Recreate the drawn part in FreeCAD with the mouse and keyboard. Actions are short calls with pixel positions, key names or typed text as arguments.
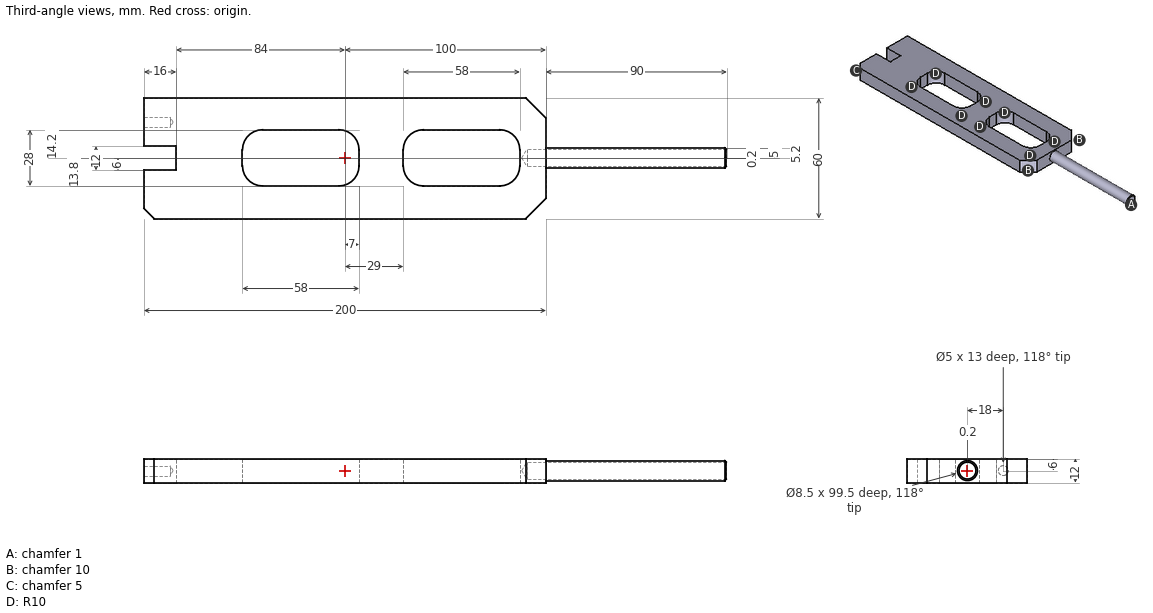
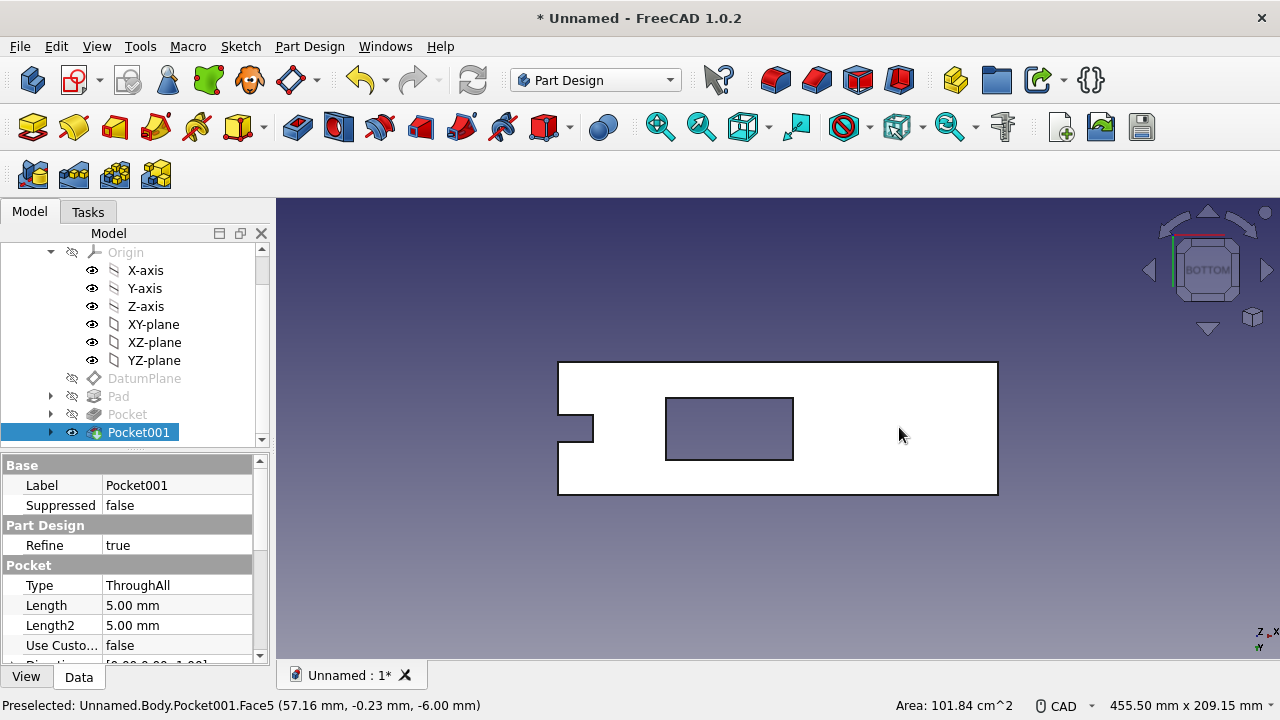
click(74, 80)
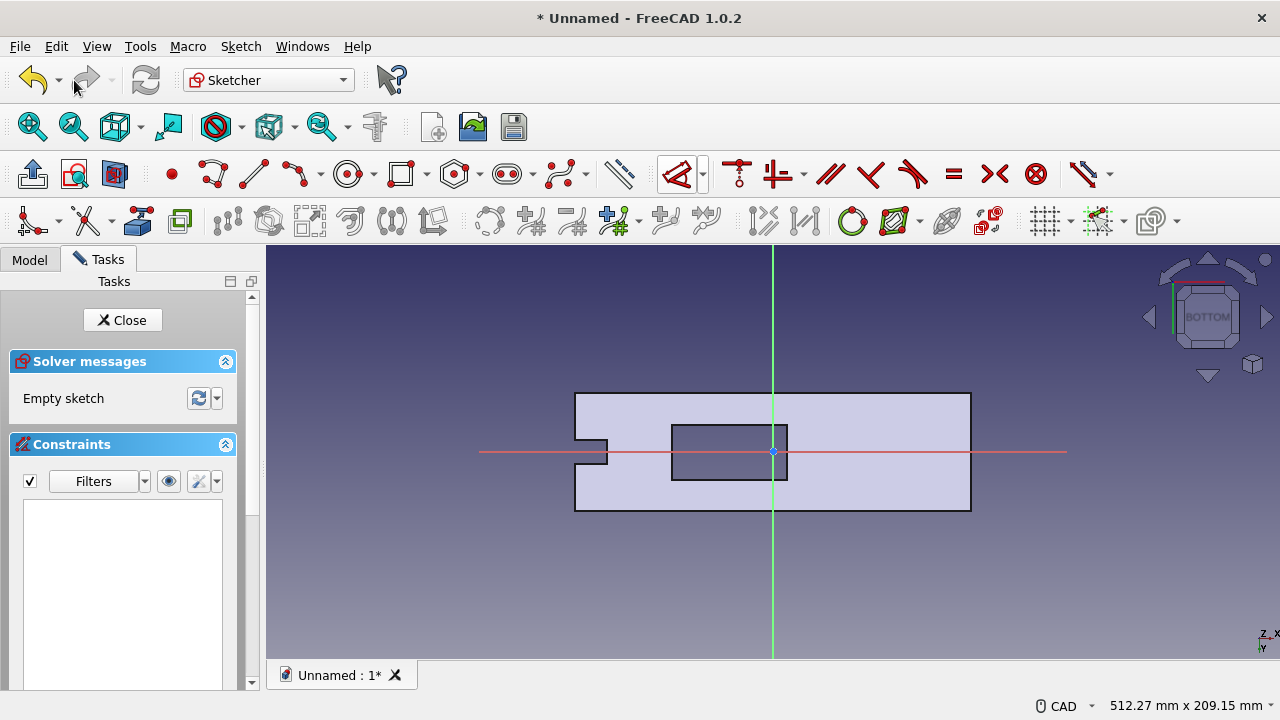
scroll(926, 453, up, 6)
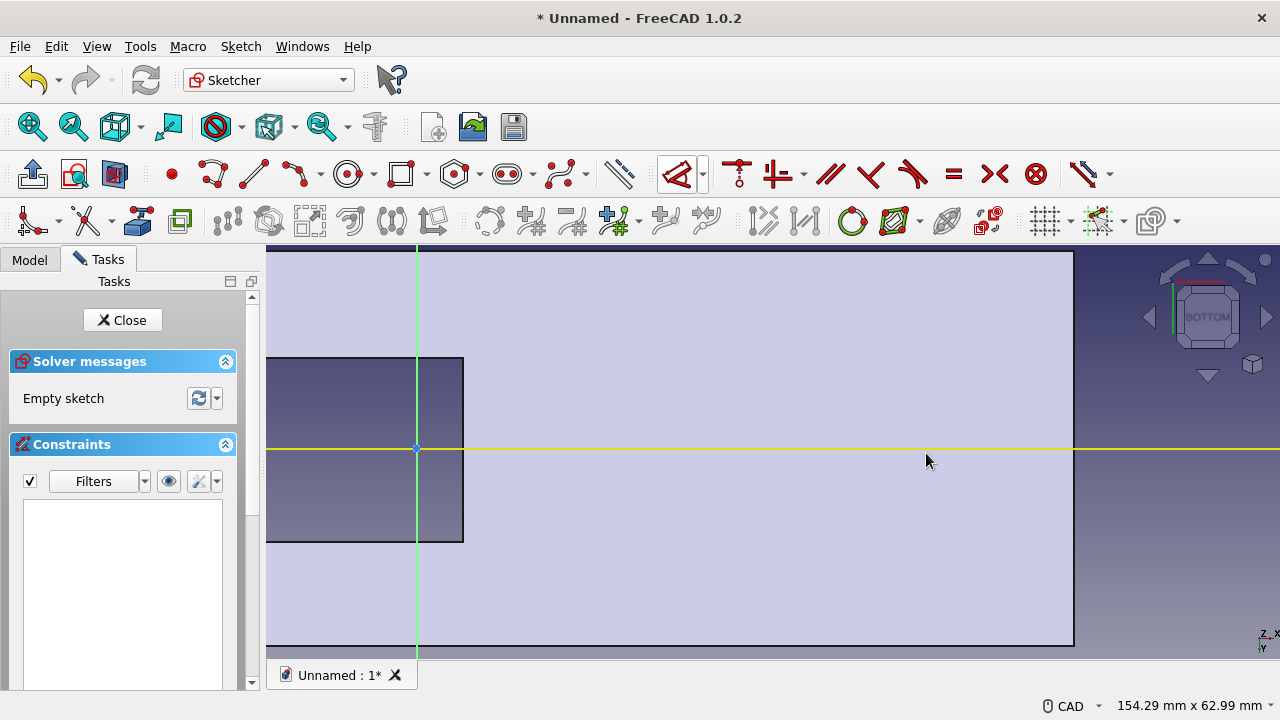
key(g)
key(r)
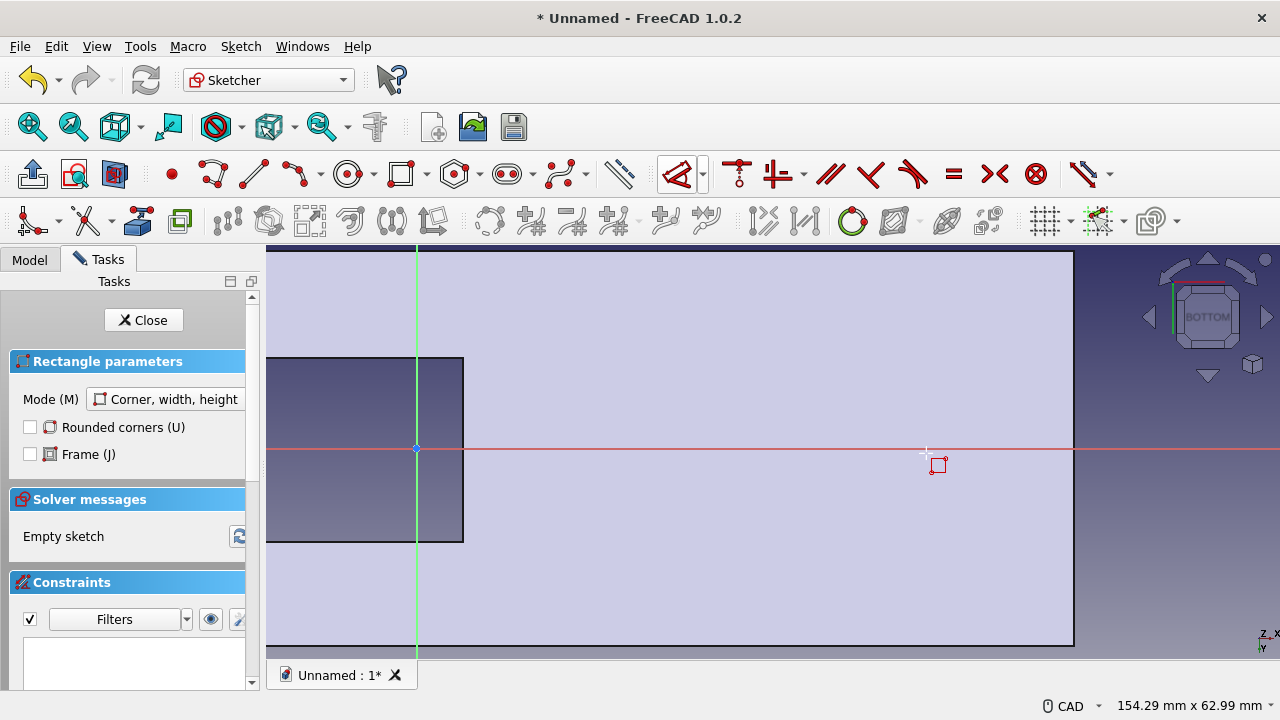
click(607, 358)
move(988, 542)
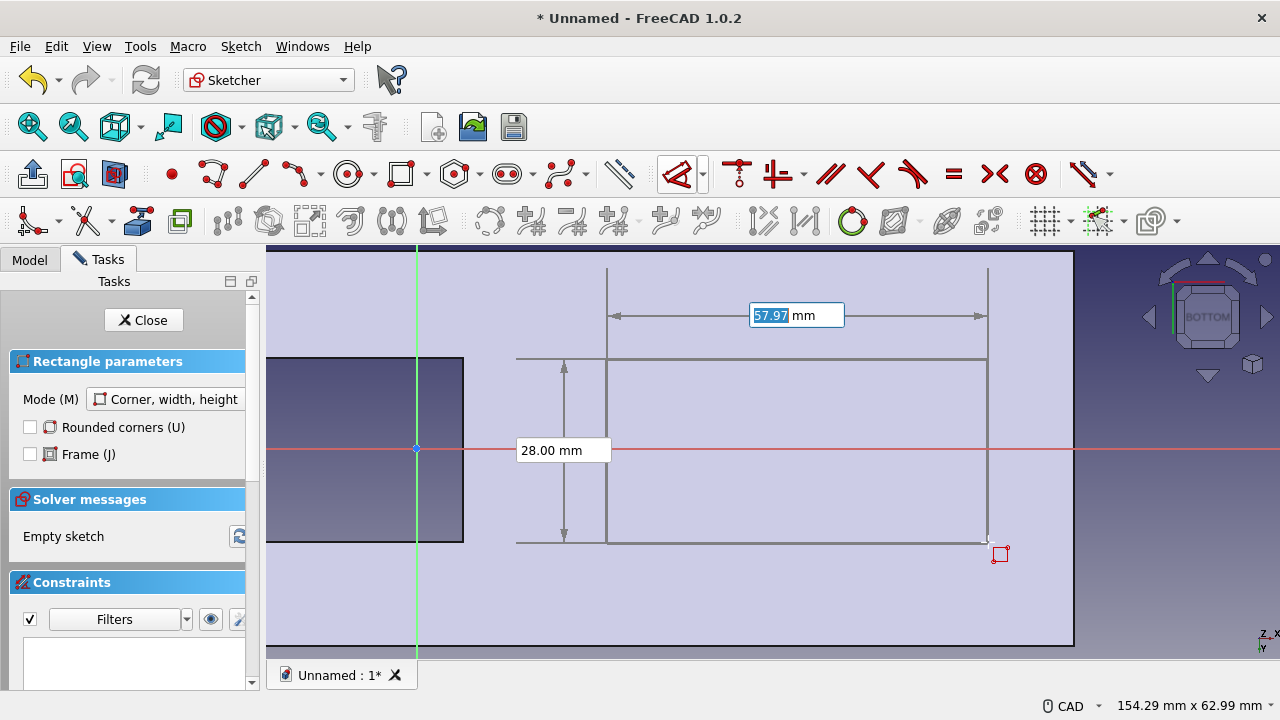
text(58)
key(Tab)
text(28)
key(Return)
key(Escape)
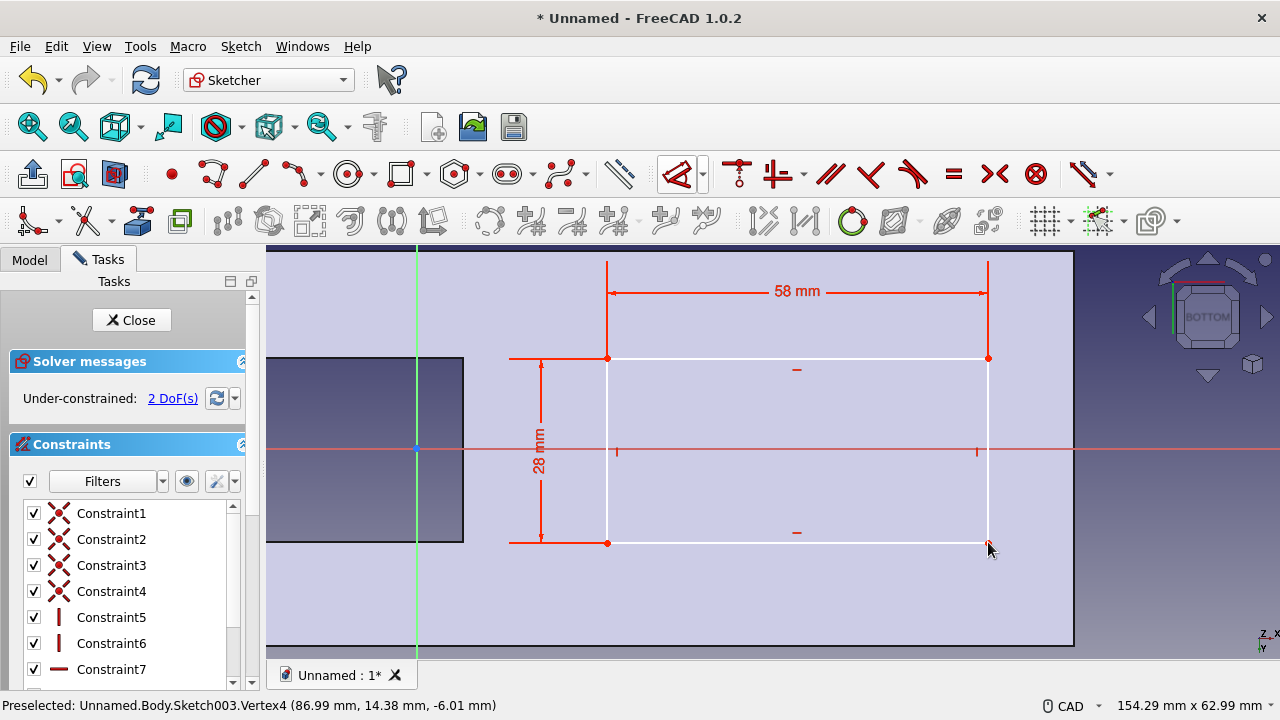
click(607, 359)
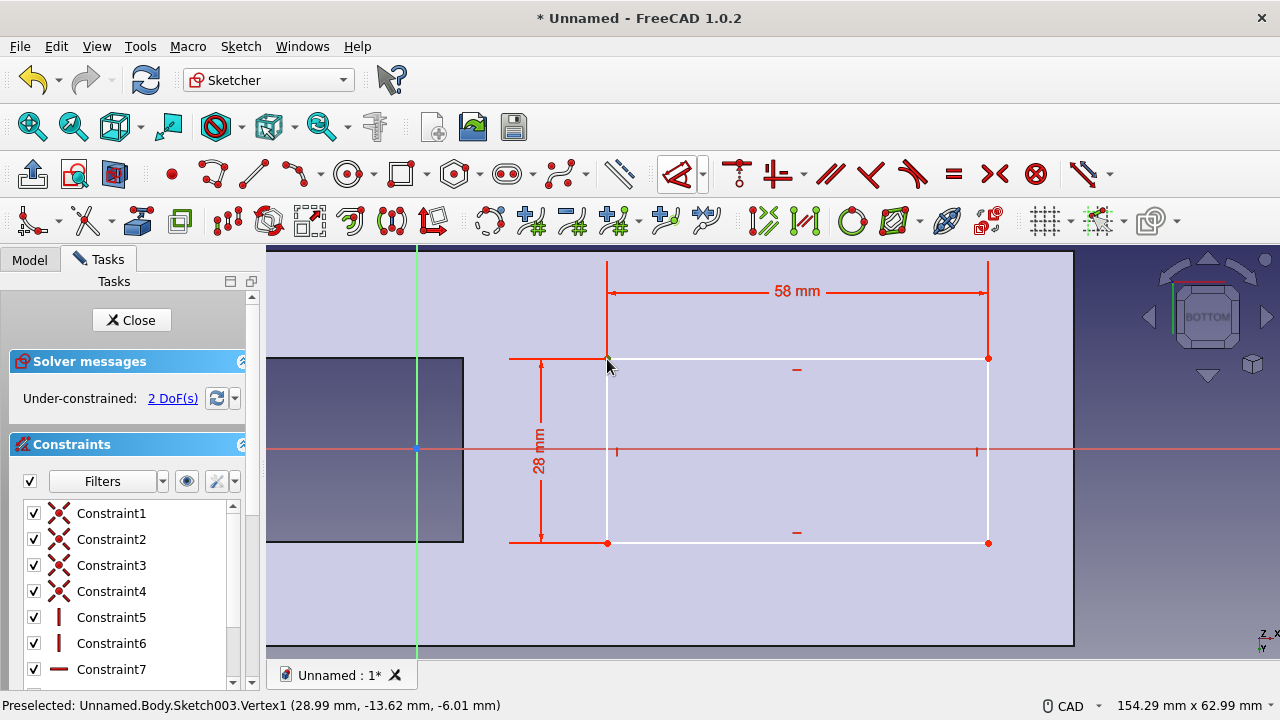
click(702, 174)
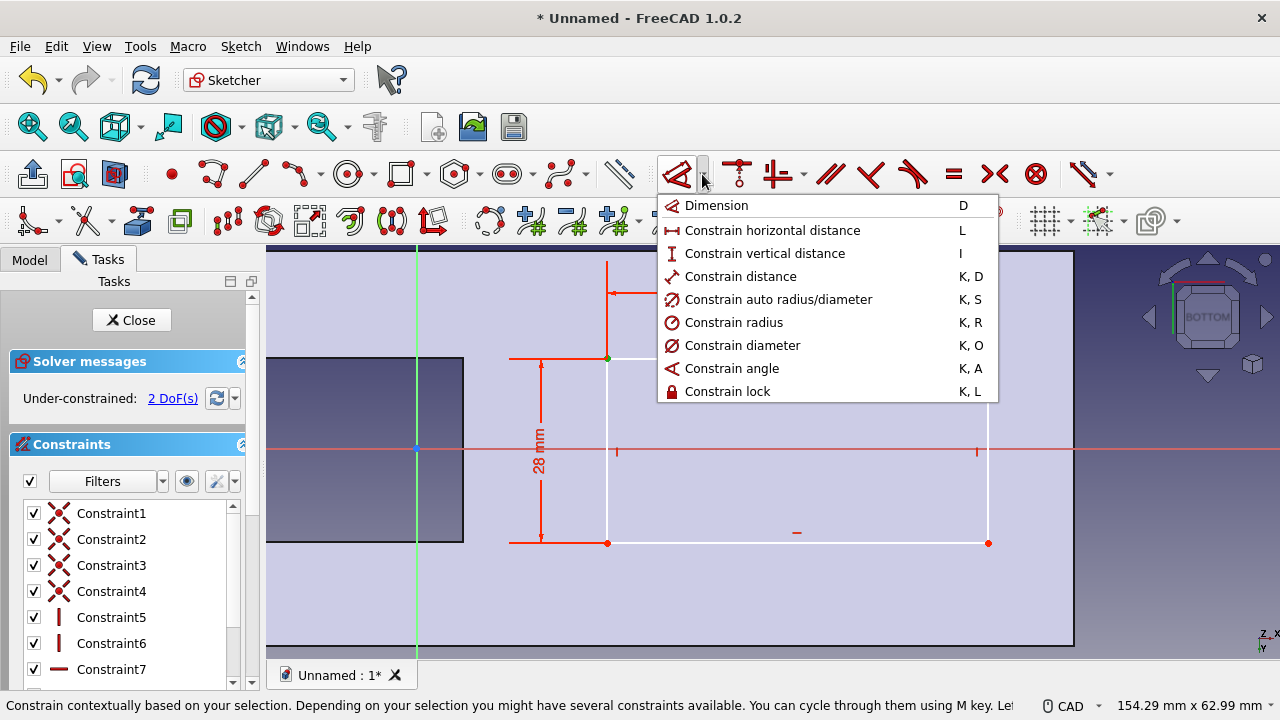
click(828, 230)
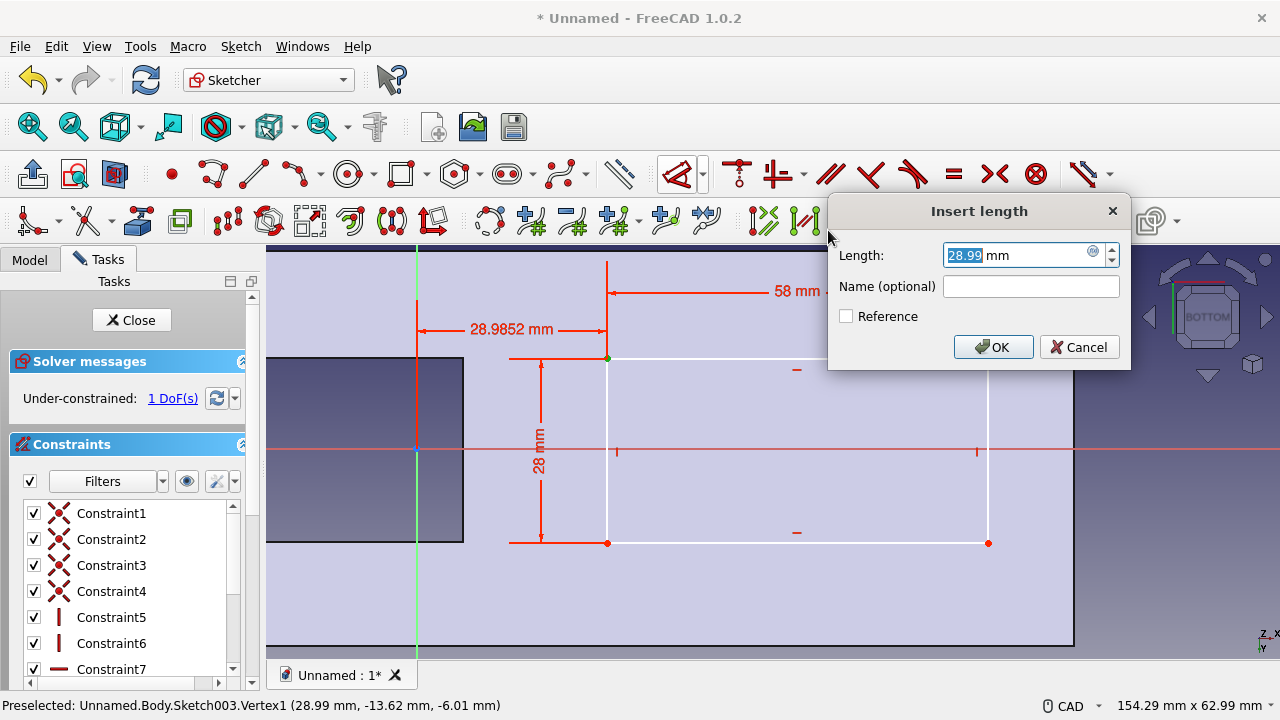
text(29)
key(Return)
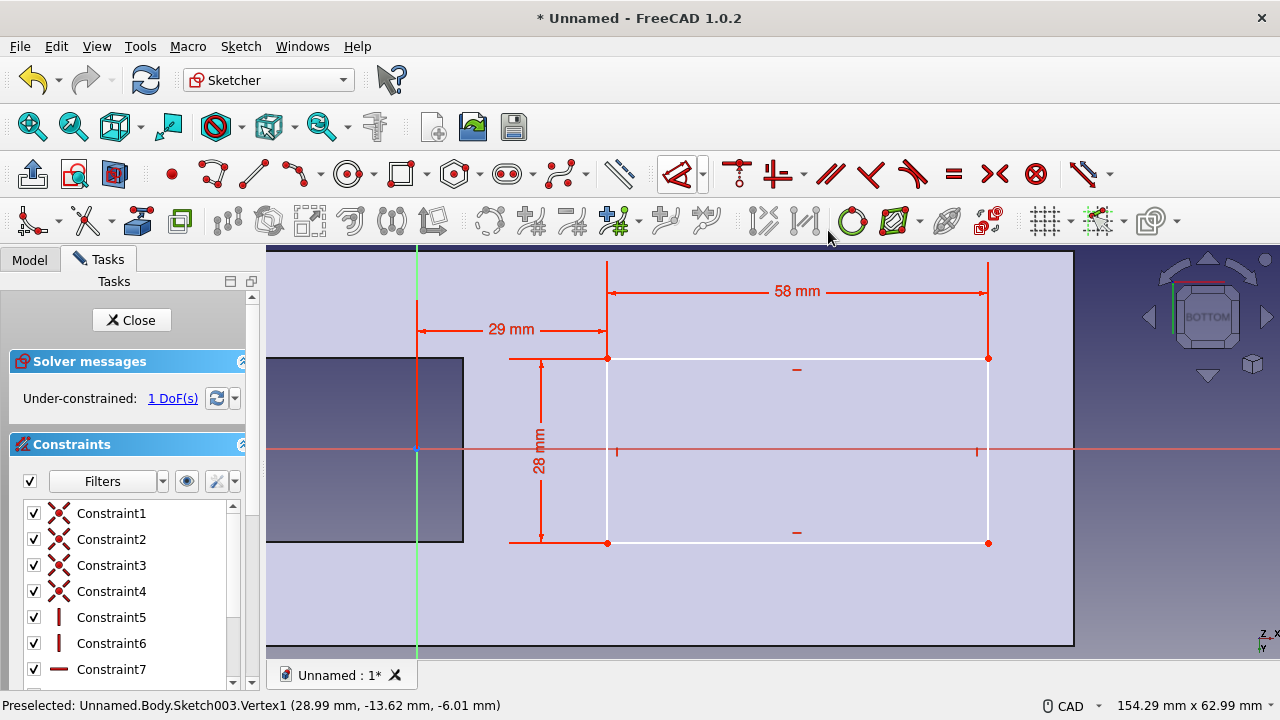
click(607, 359)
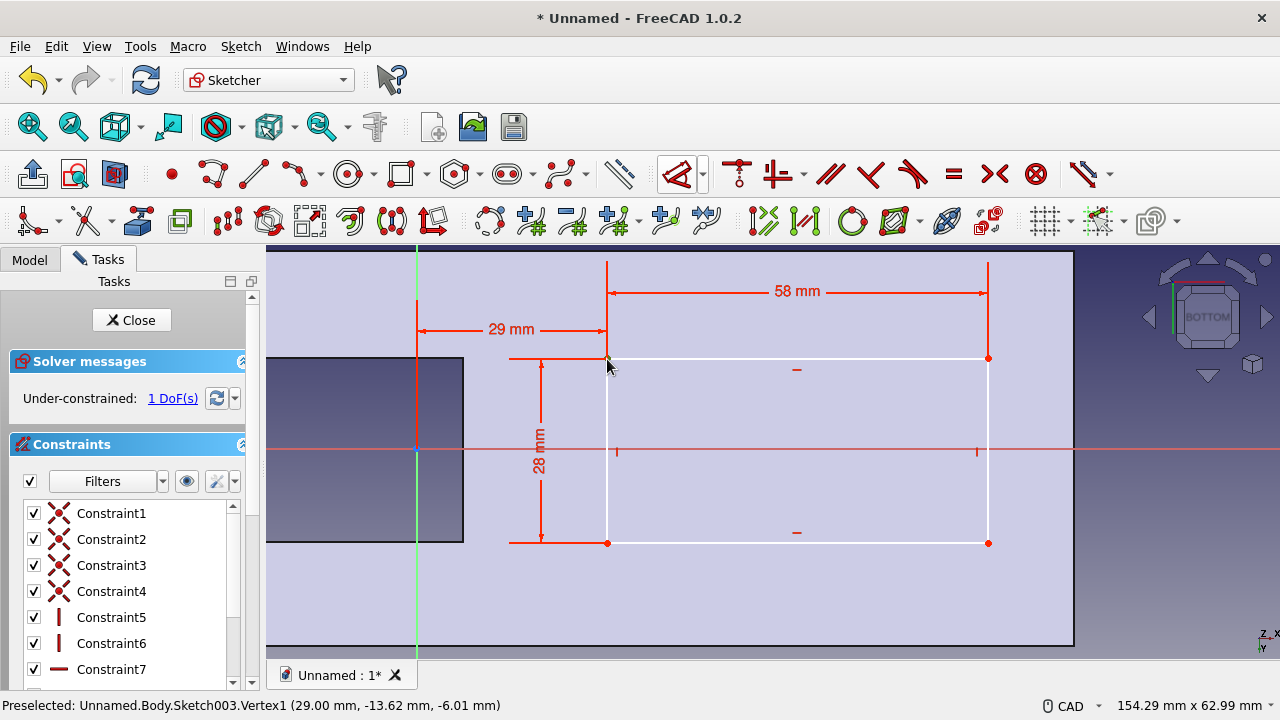
key(i)